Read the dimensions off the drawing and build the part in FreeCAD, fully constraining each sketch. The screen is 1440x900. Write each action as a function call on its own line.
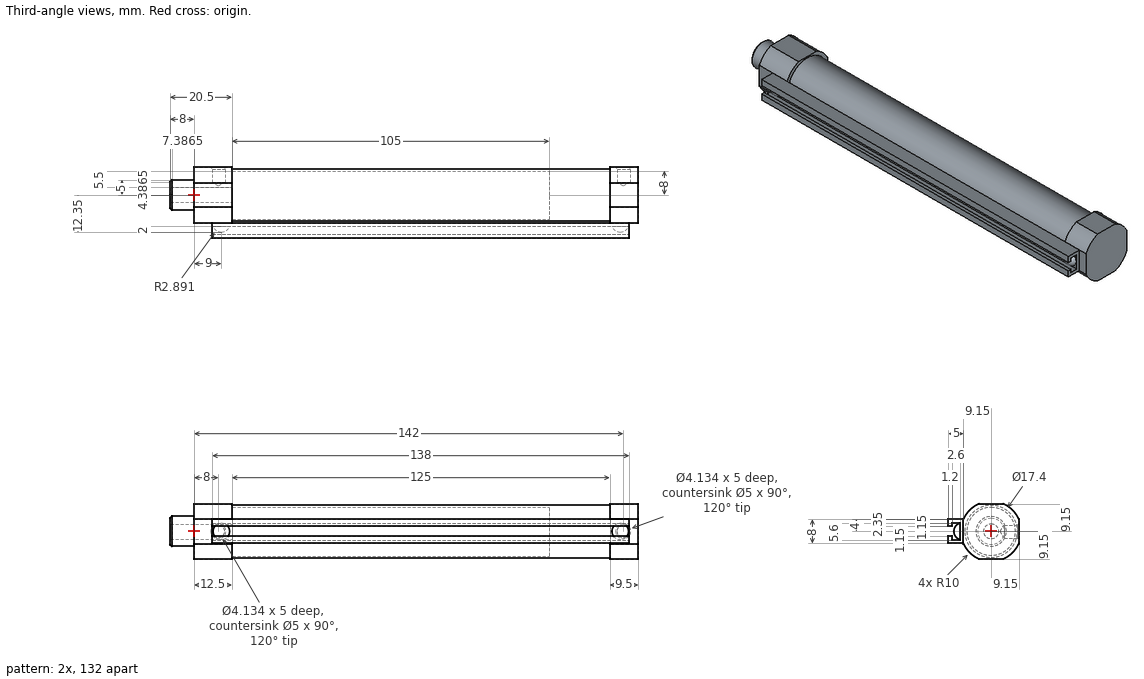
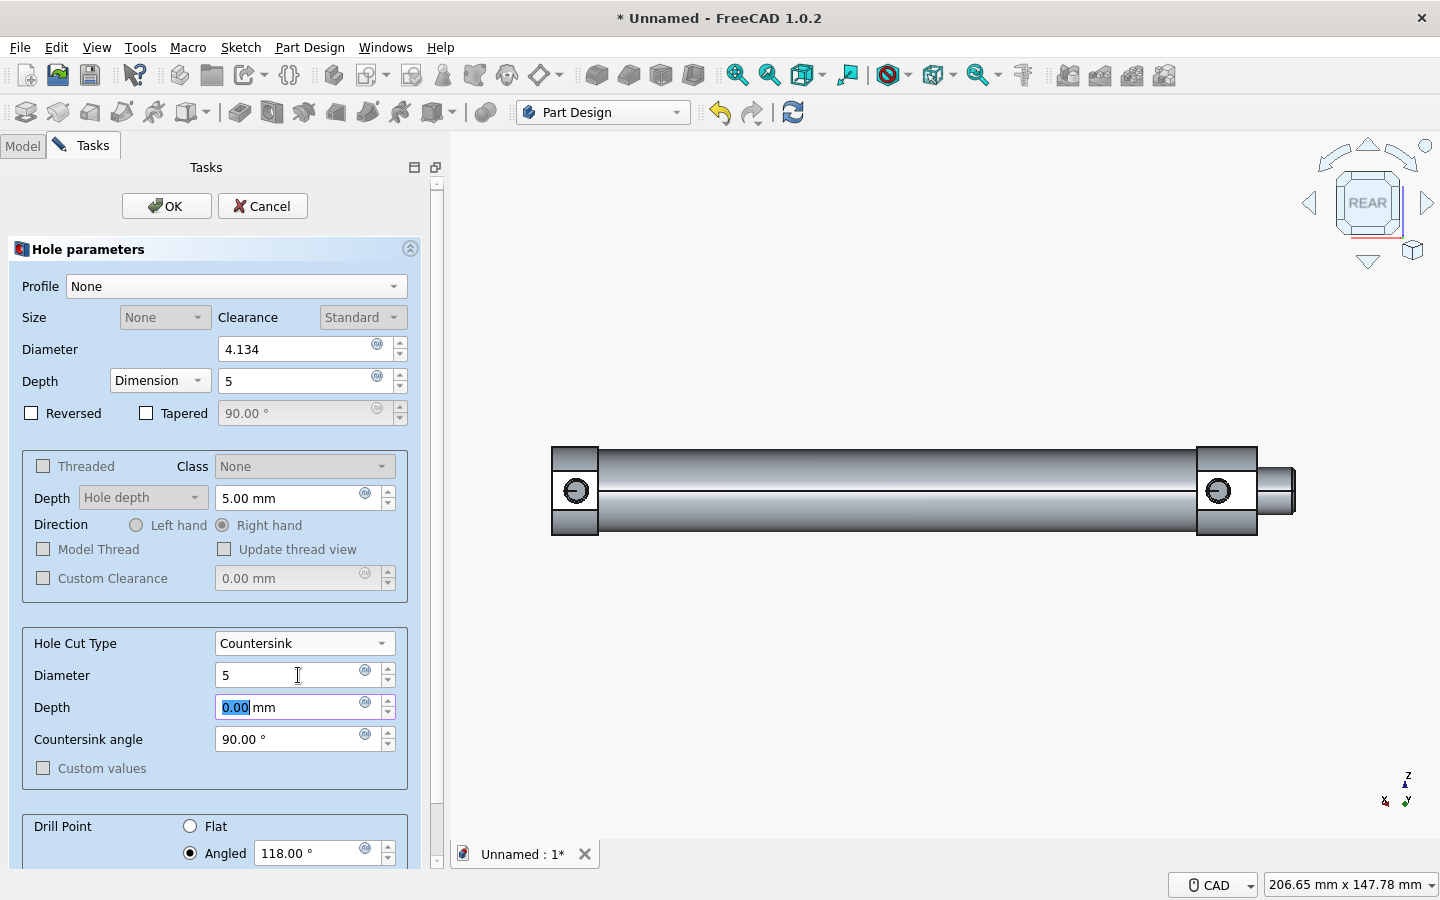
triple_click(317, 853)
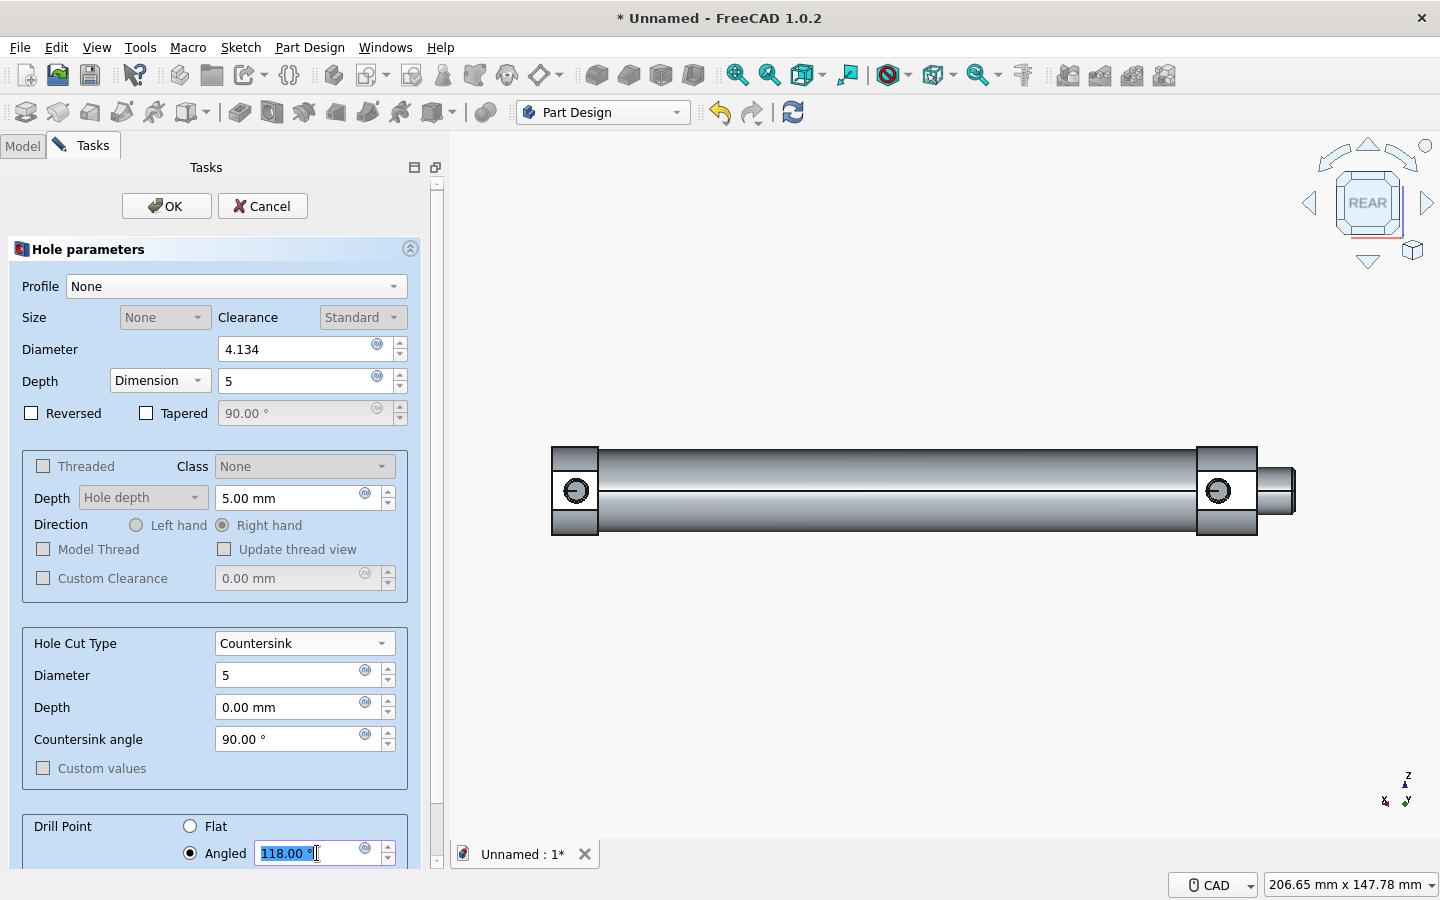
text(120)
key(Tab)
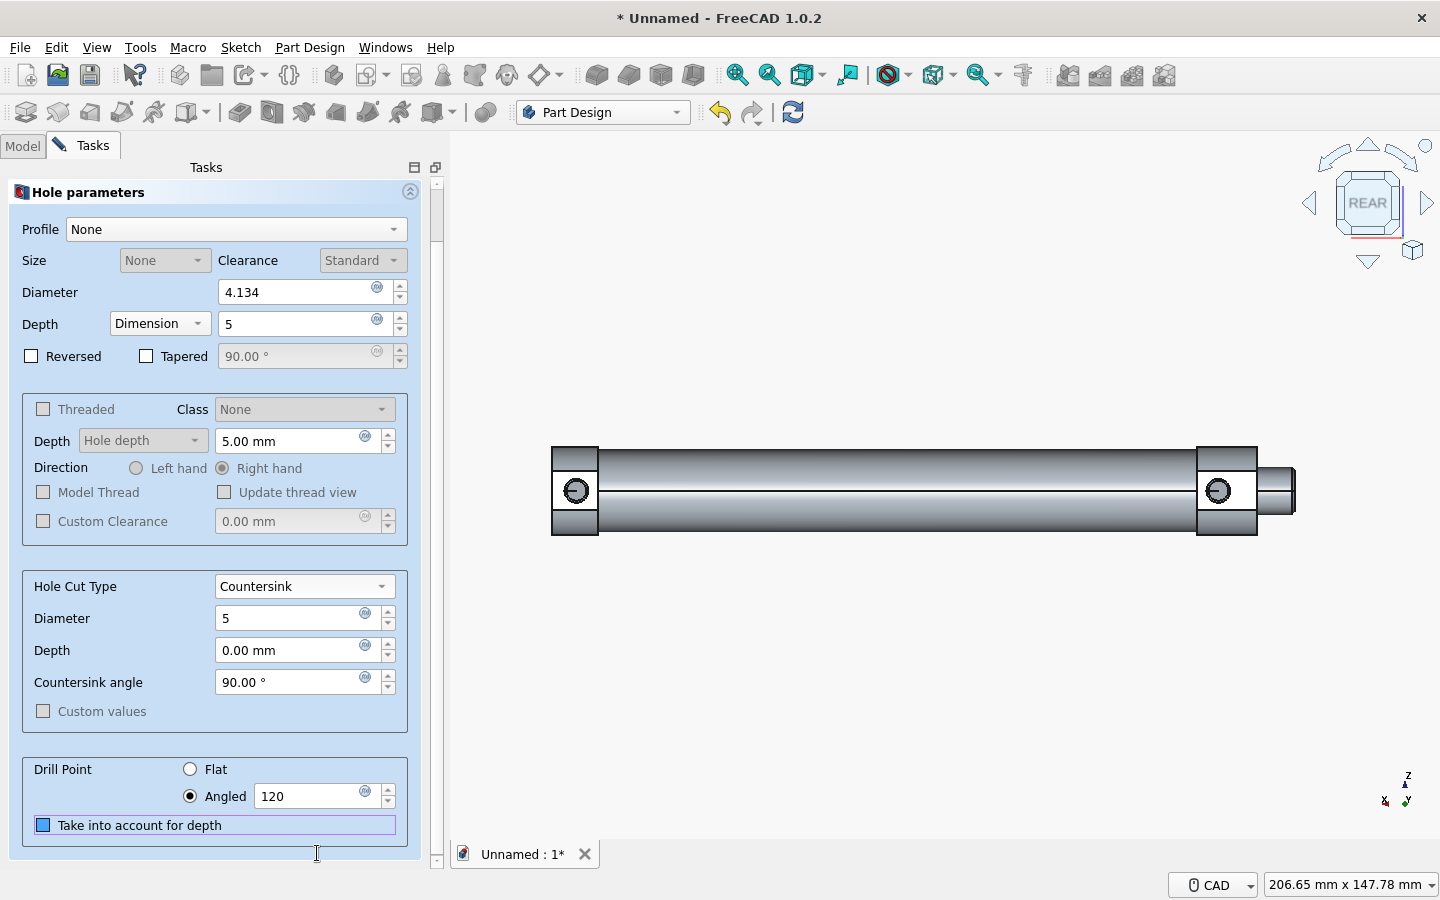
scroll(437, 522, up, 2)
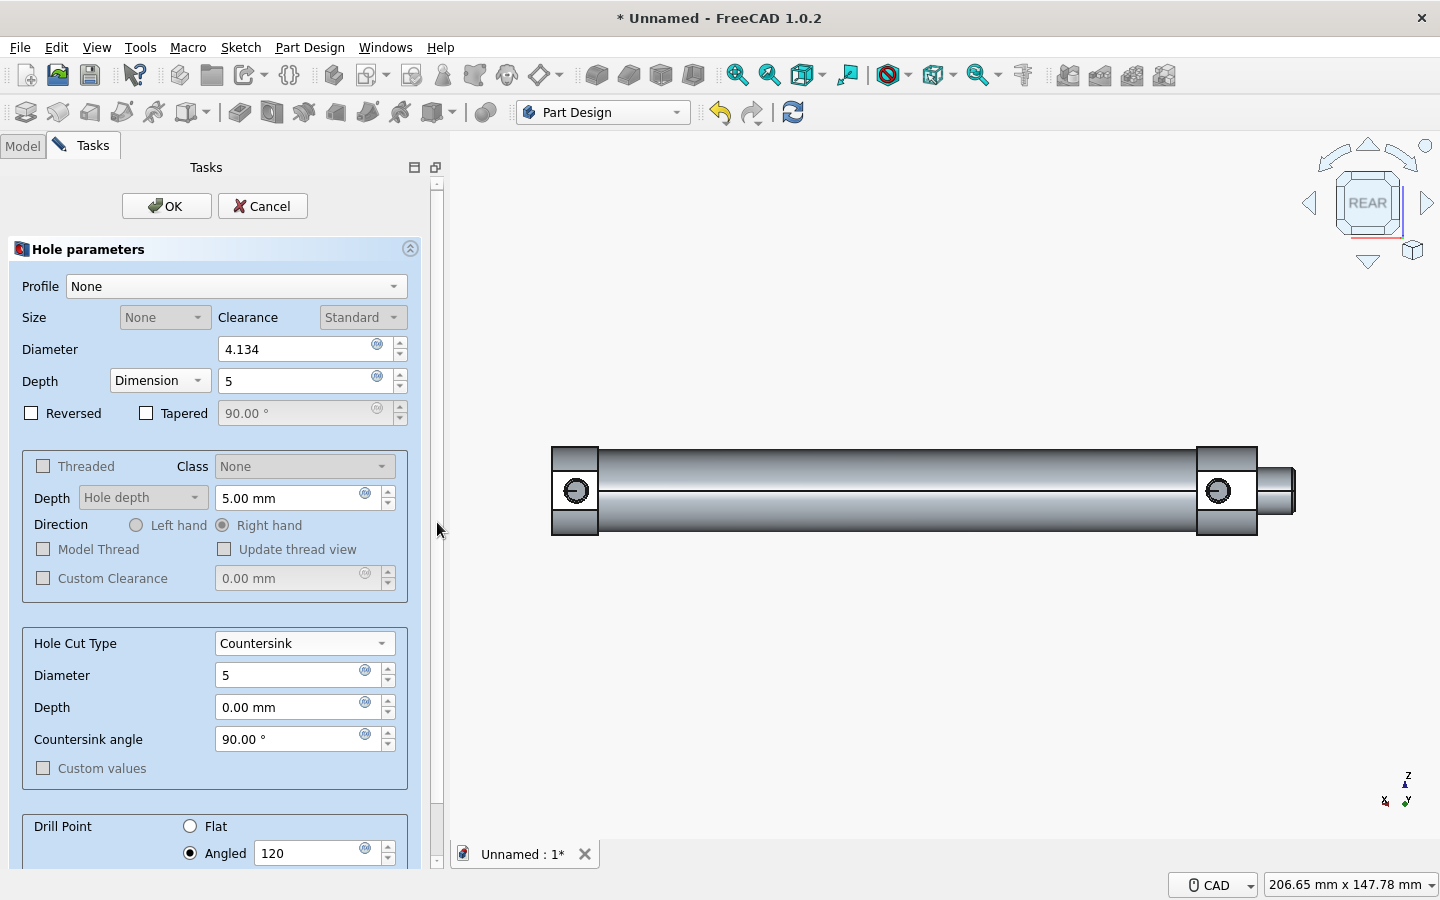
click(167, 206)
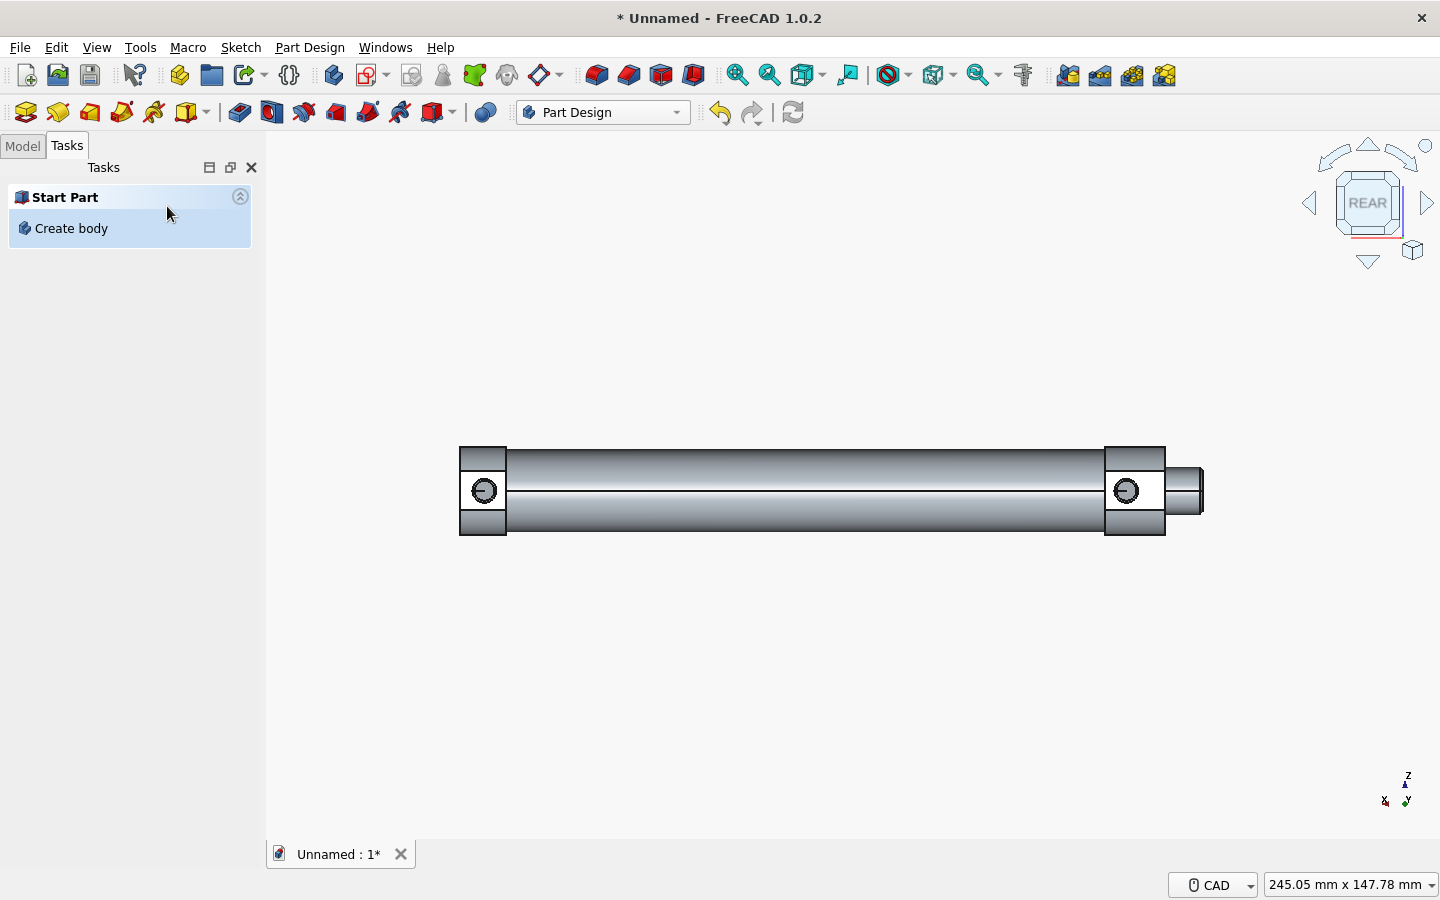
click(366, 76)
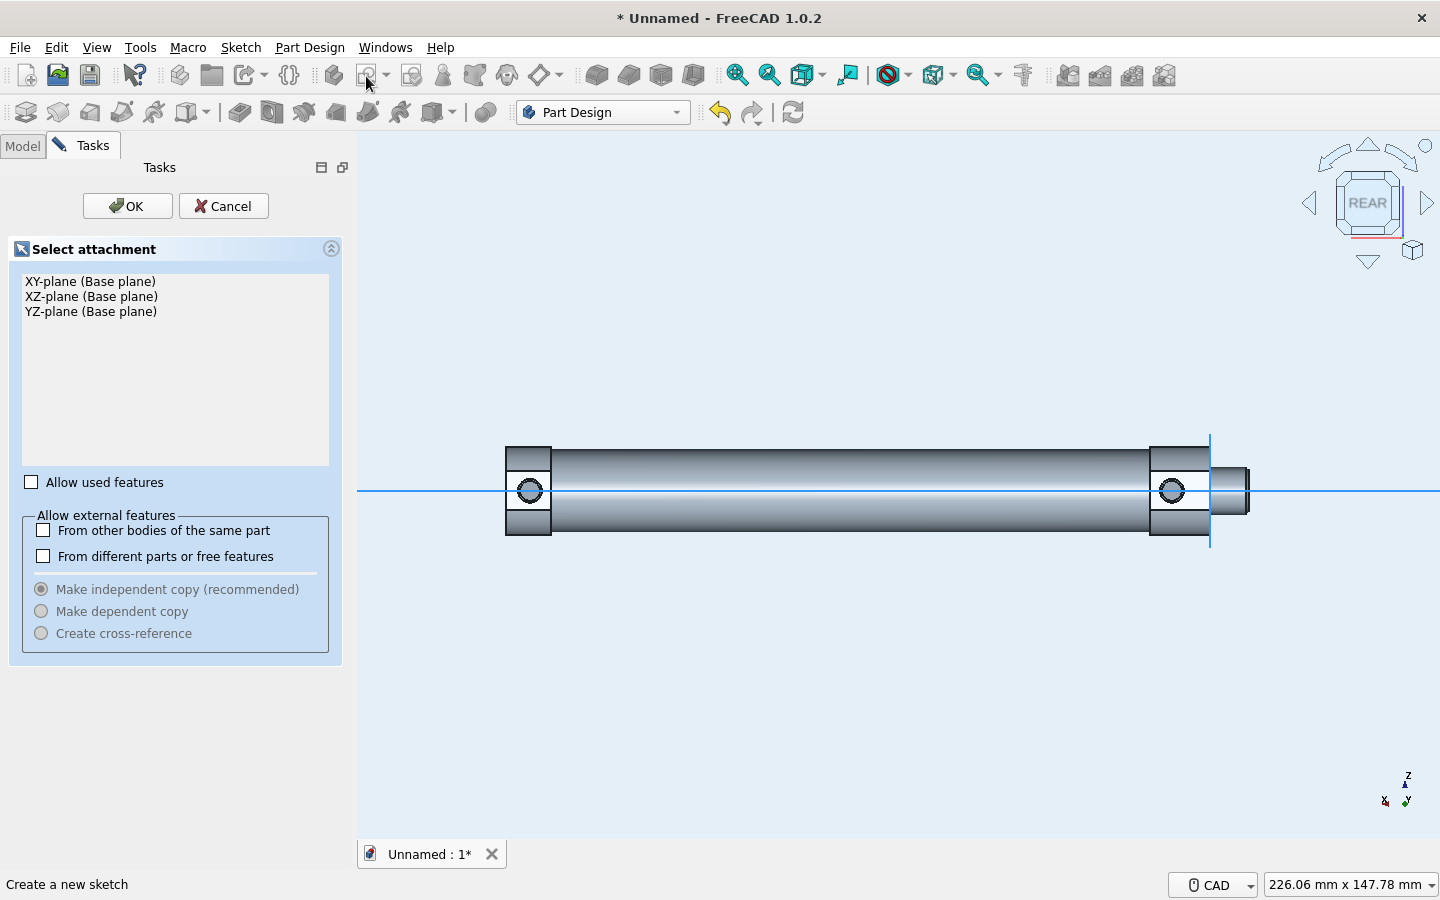
click(82, 282)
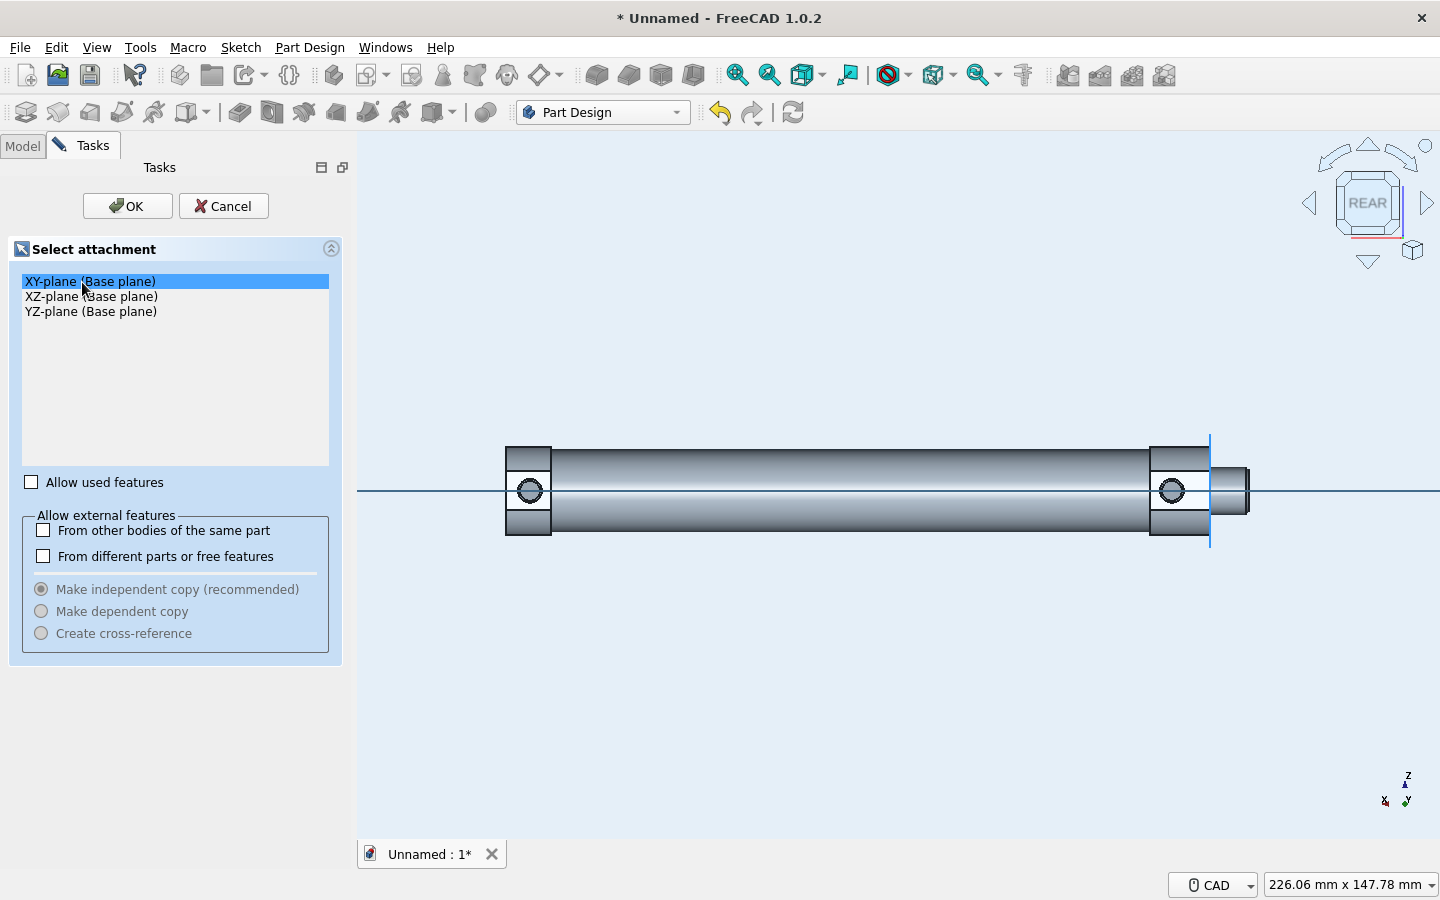
click(128, 206)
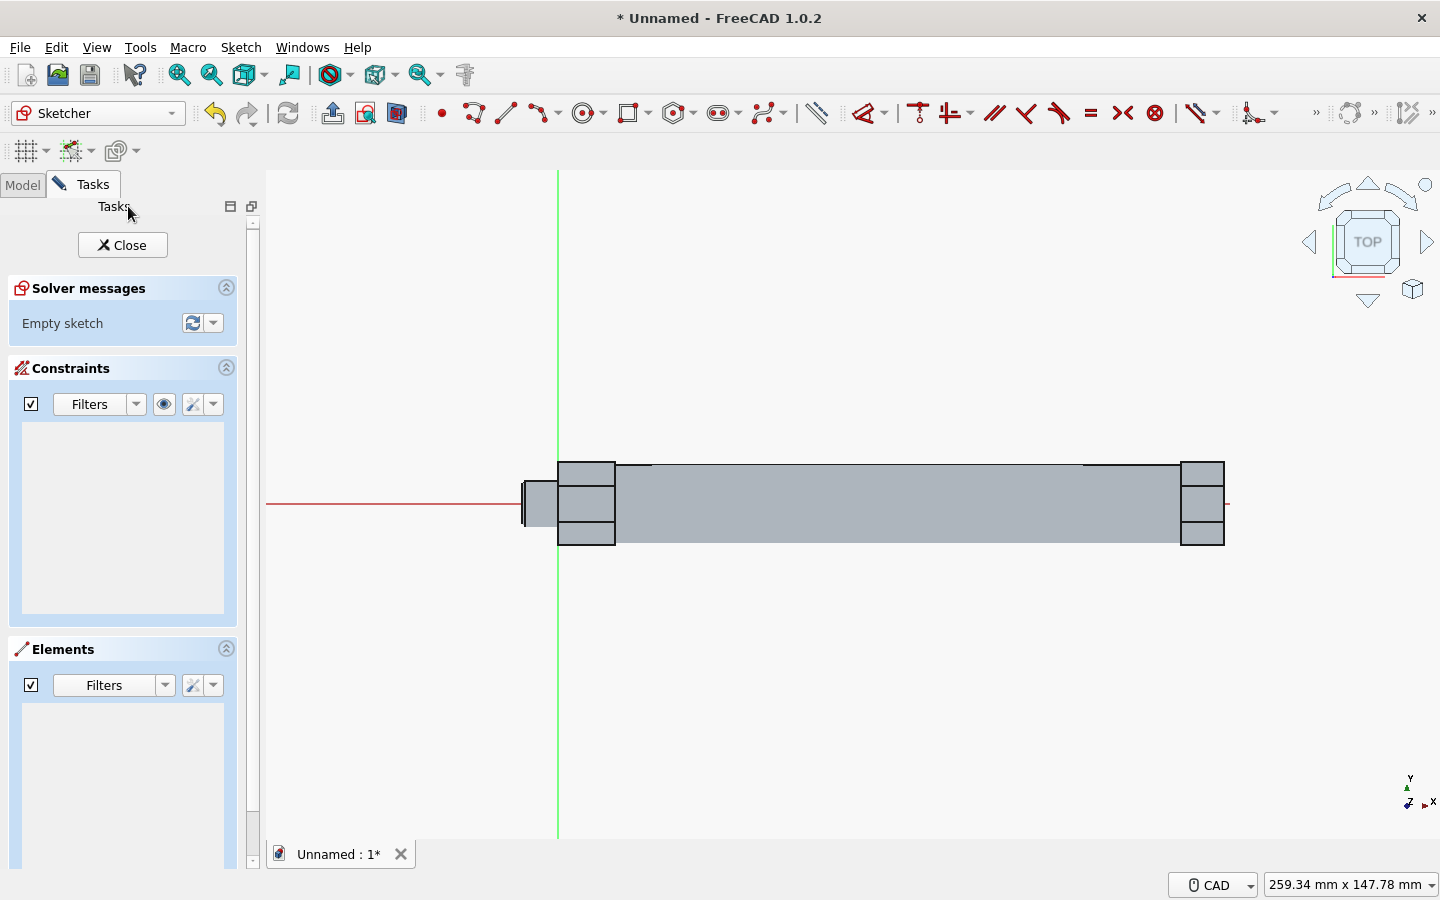
click(398, 114)